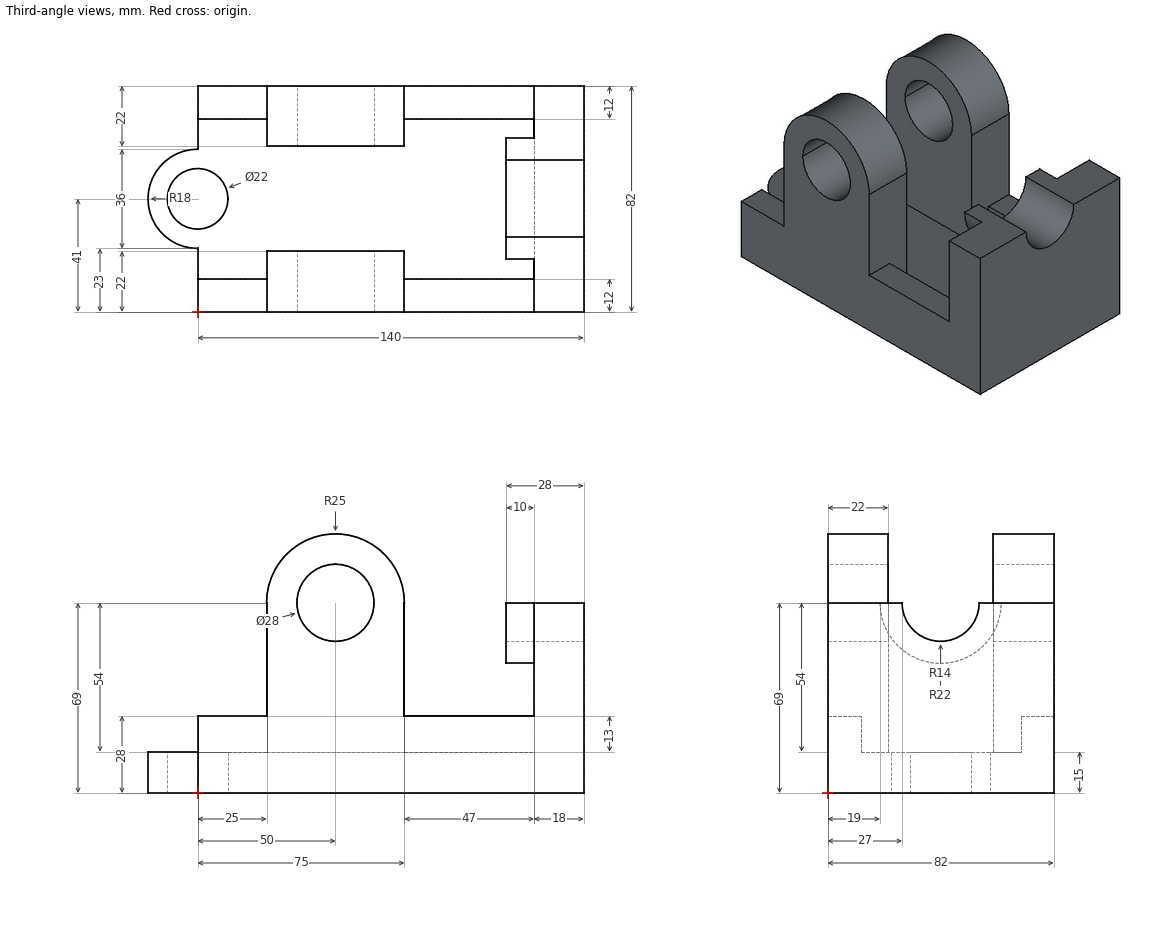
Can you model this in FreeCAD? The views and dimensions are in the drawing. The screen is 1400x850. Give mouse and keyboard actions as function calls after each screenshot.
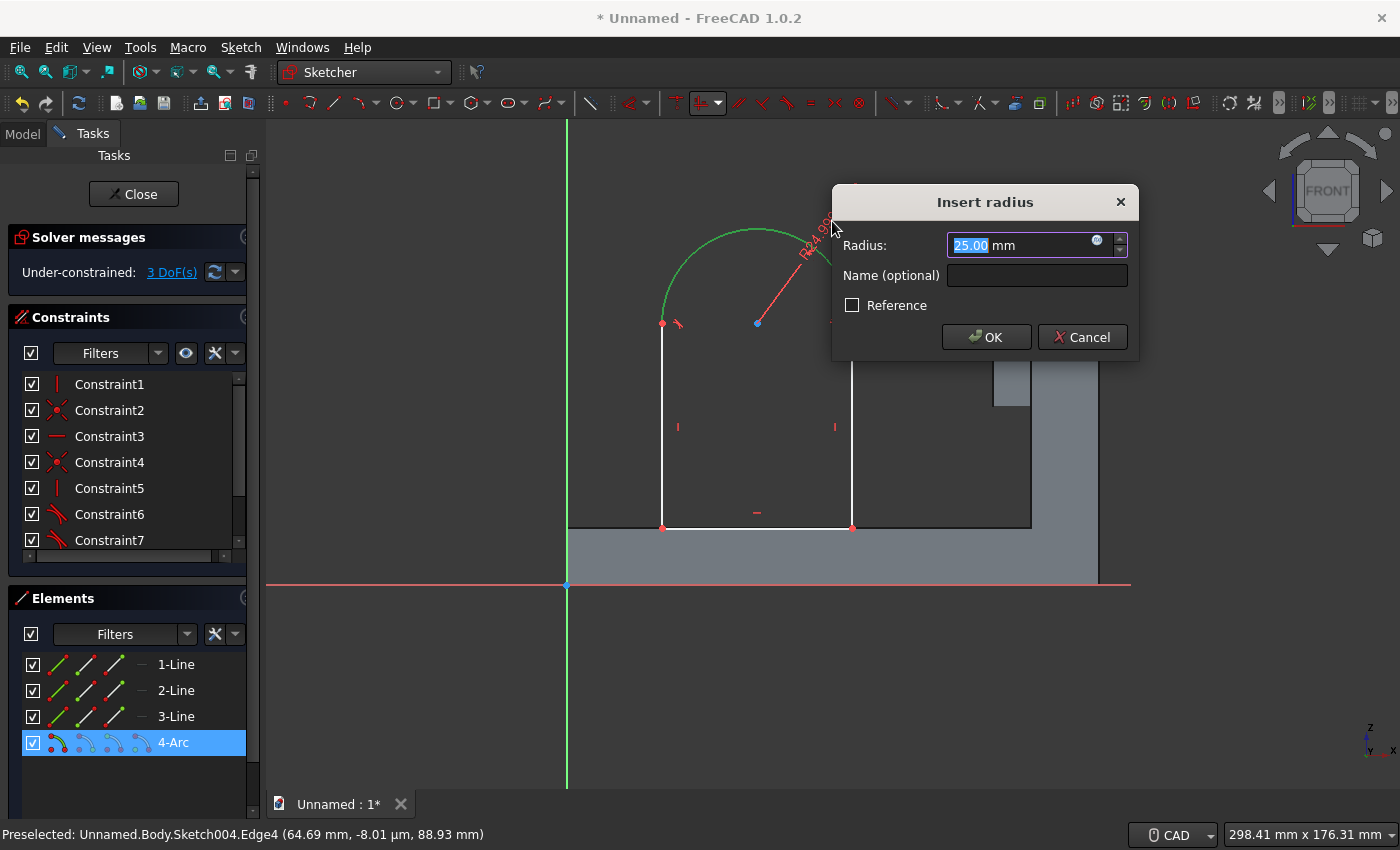
text(25)
key(Return)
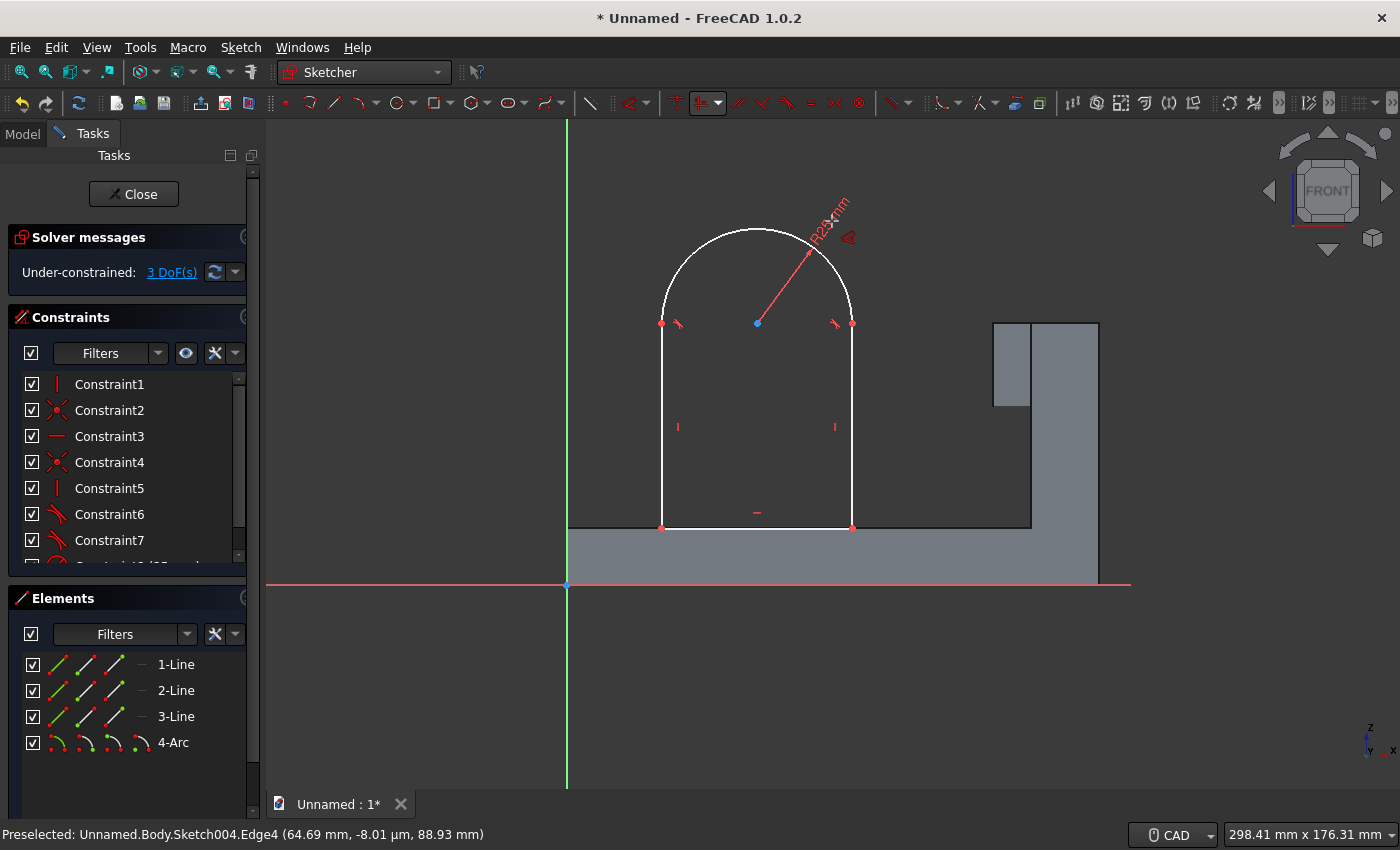
click(662, 385)
click(628, 426)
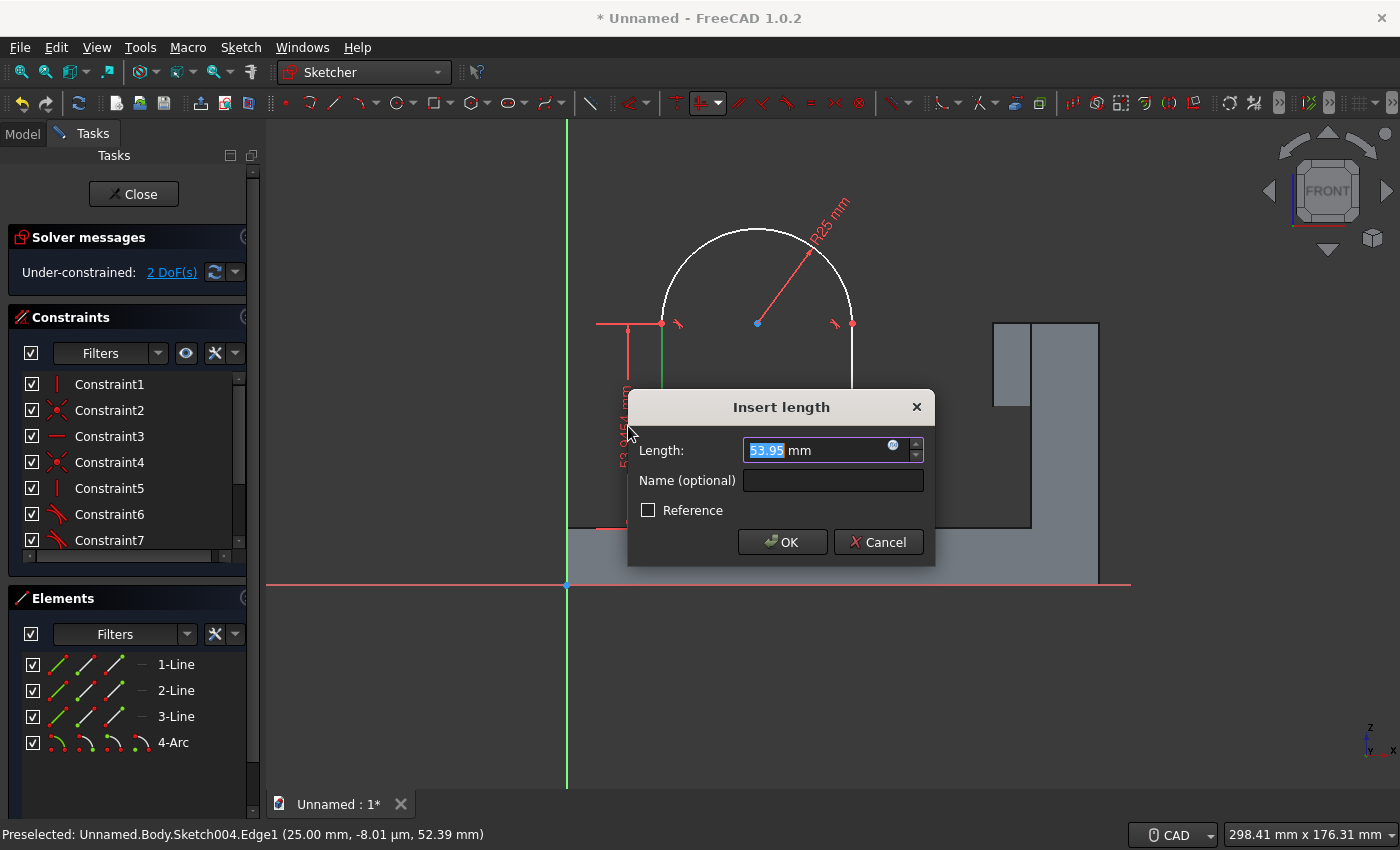
text(54)
key(Return)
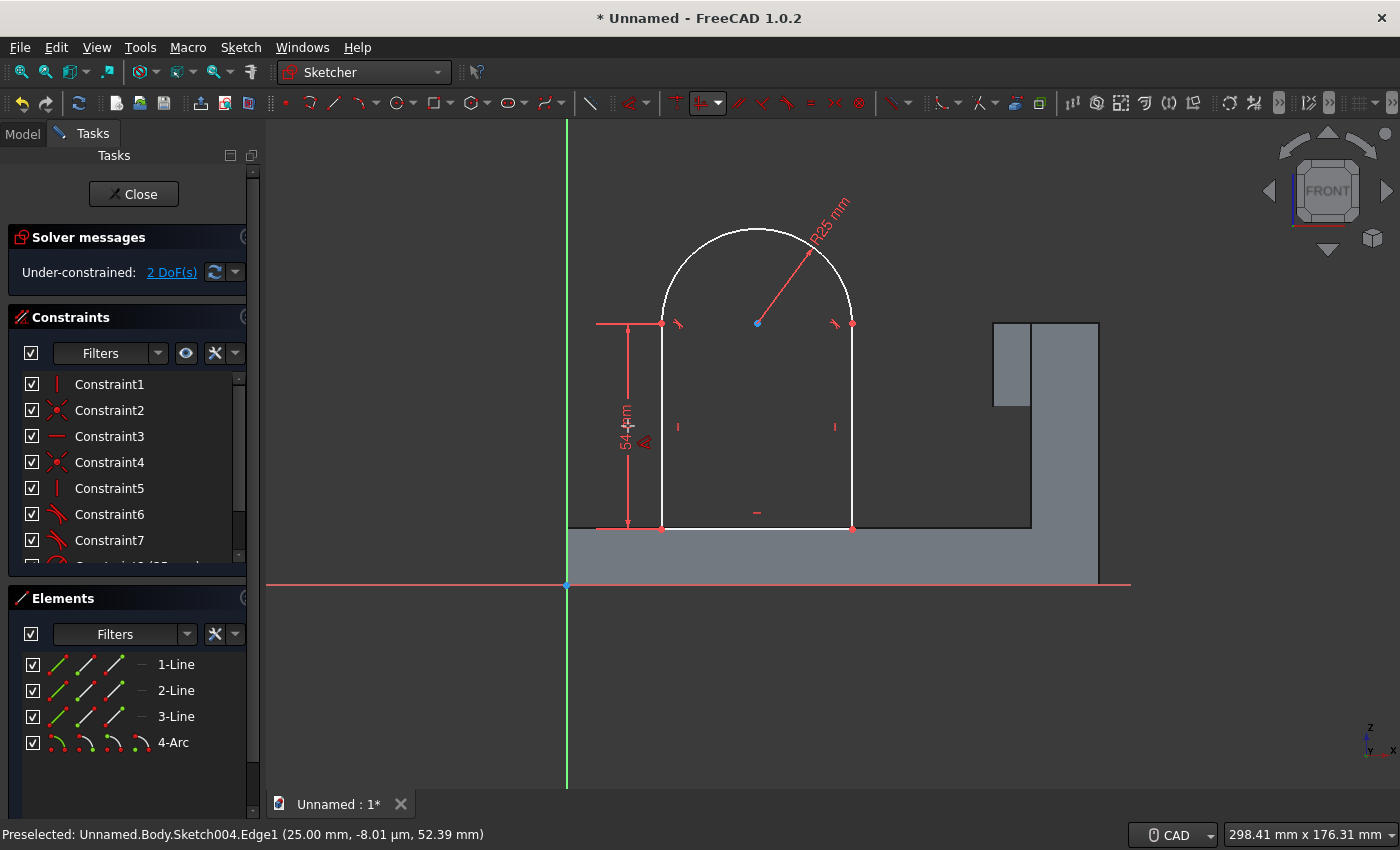
click(662, 324)
click(614, 619)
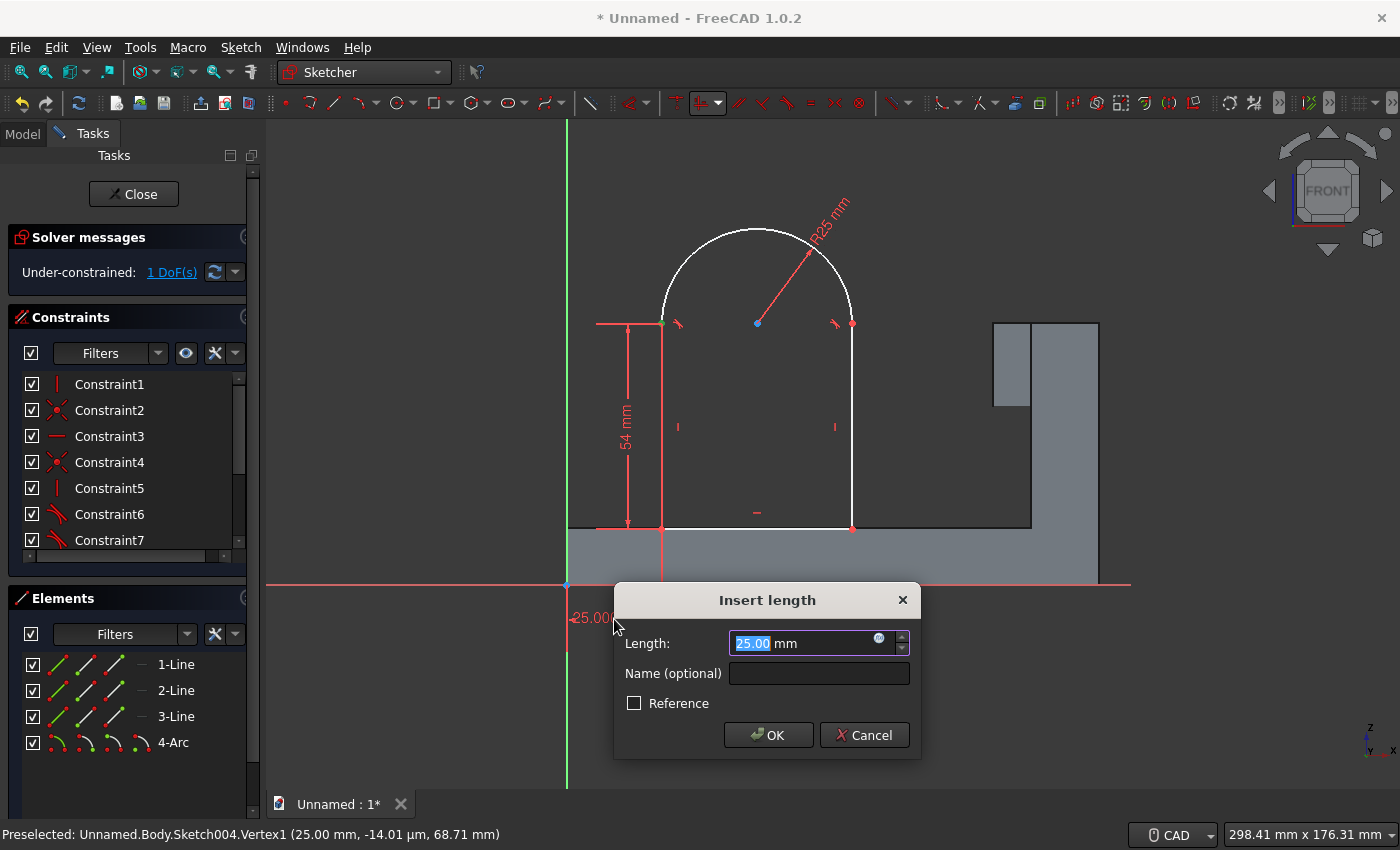
text(25)
key(Return)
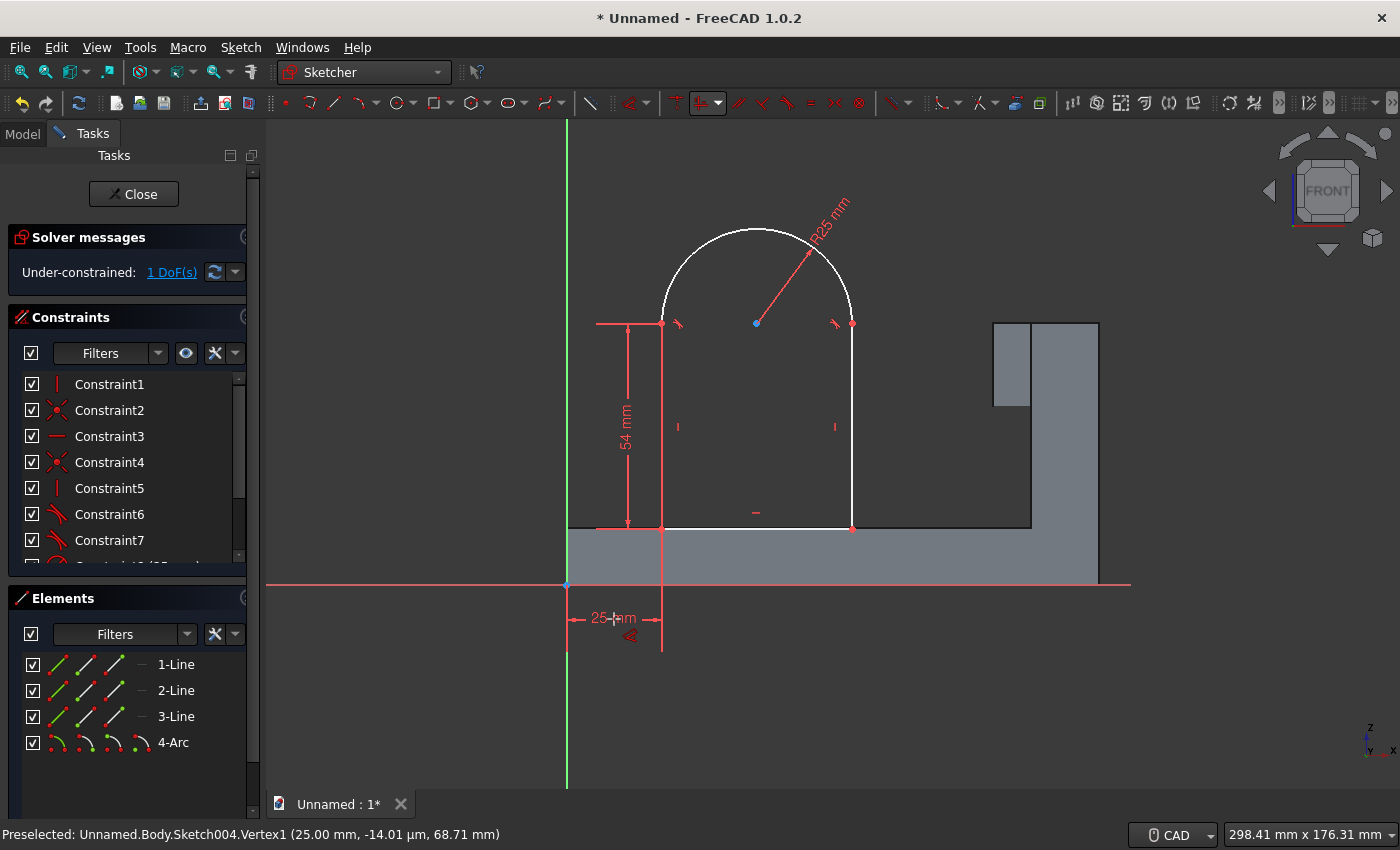
click(662, 324)
click(533, 455)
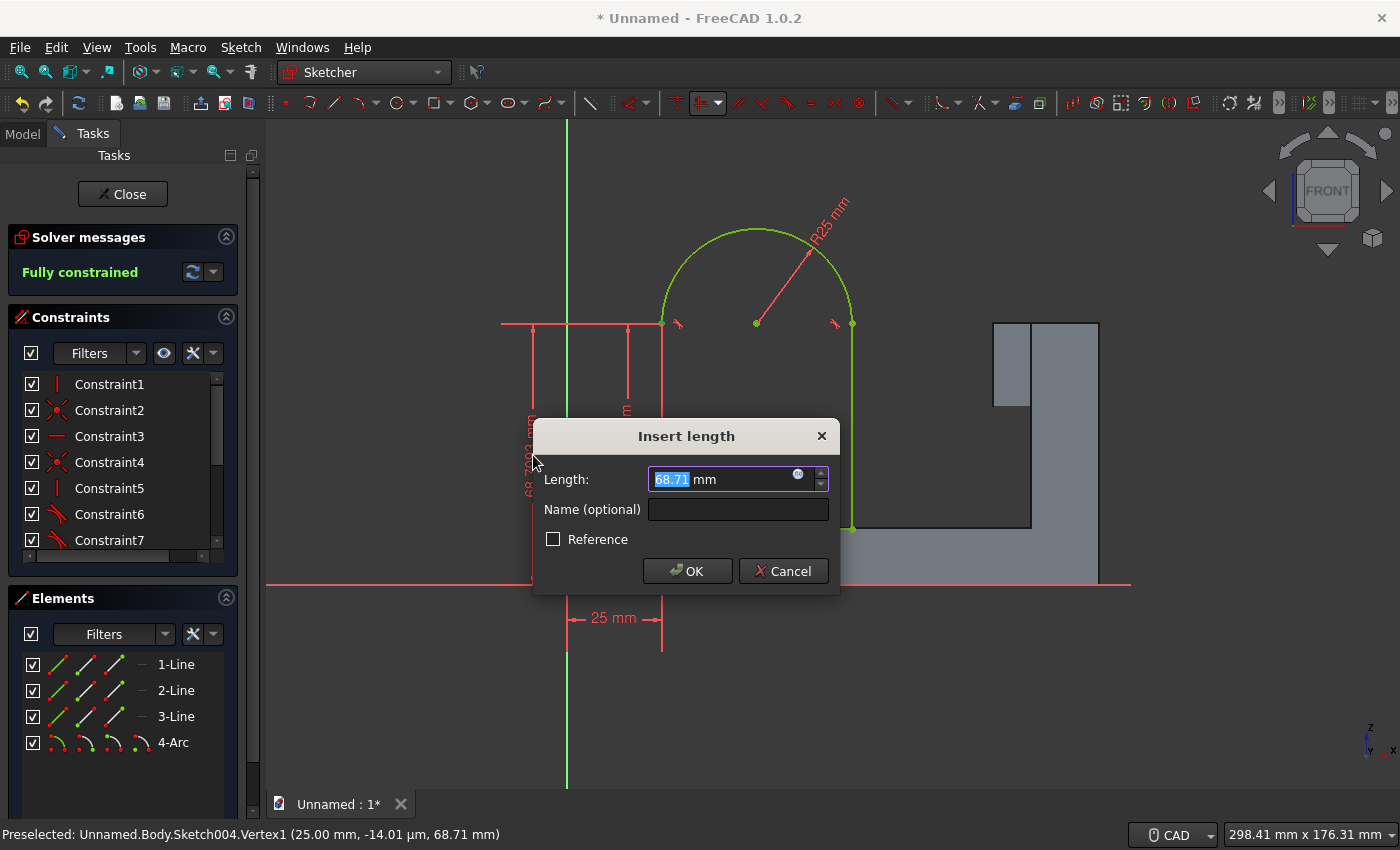
text(69)
key(Return)
key(Escape)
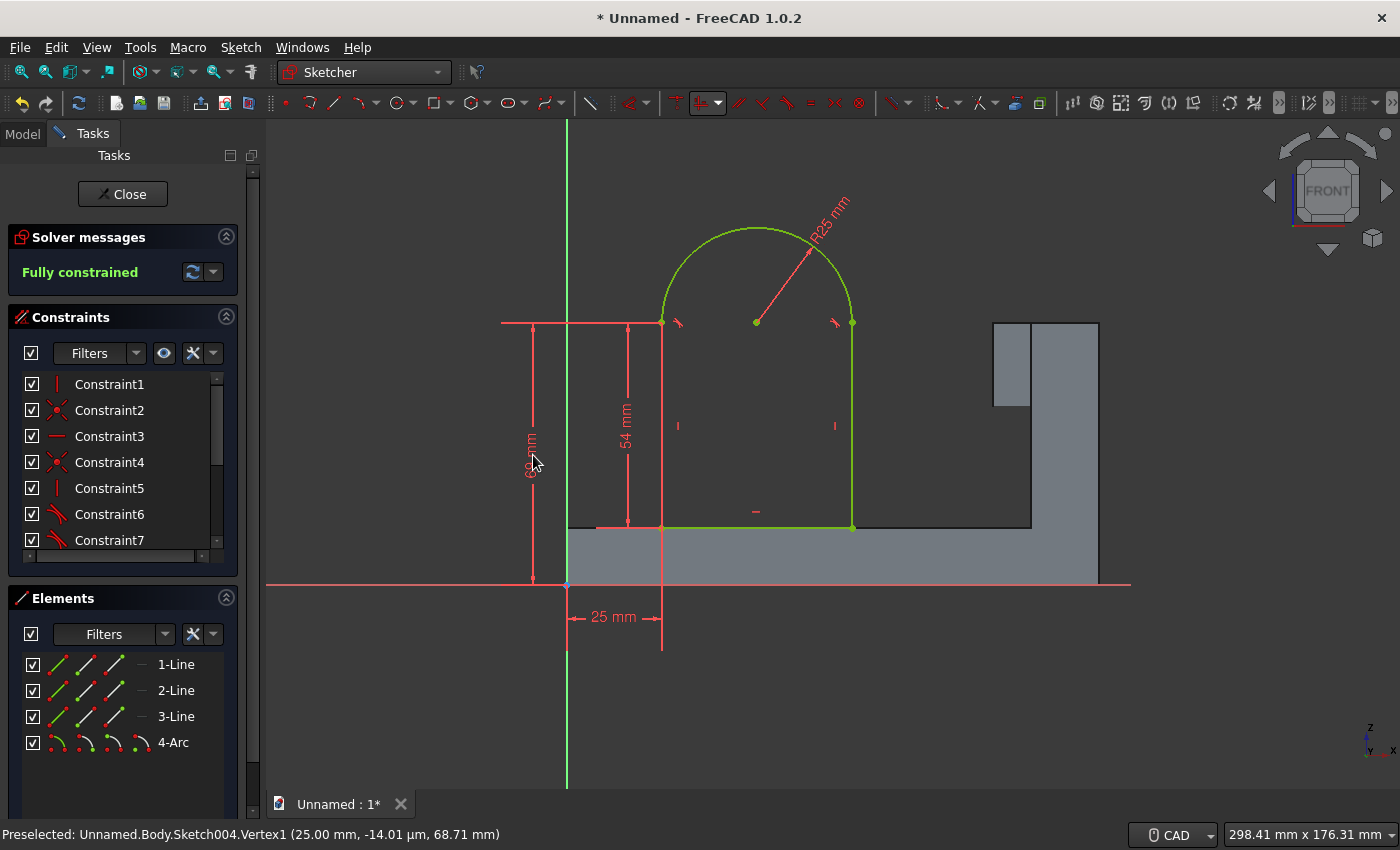
click(123, 194)